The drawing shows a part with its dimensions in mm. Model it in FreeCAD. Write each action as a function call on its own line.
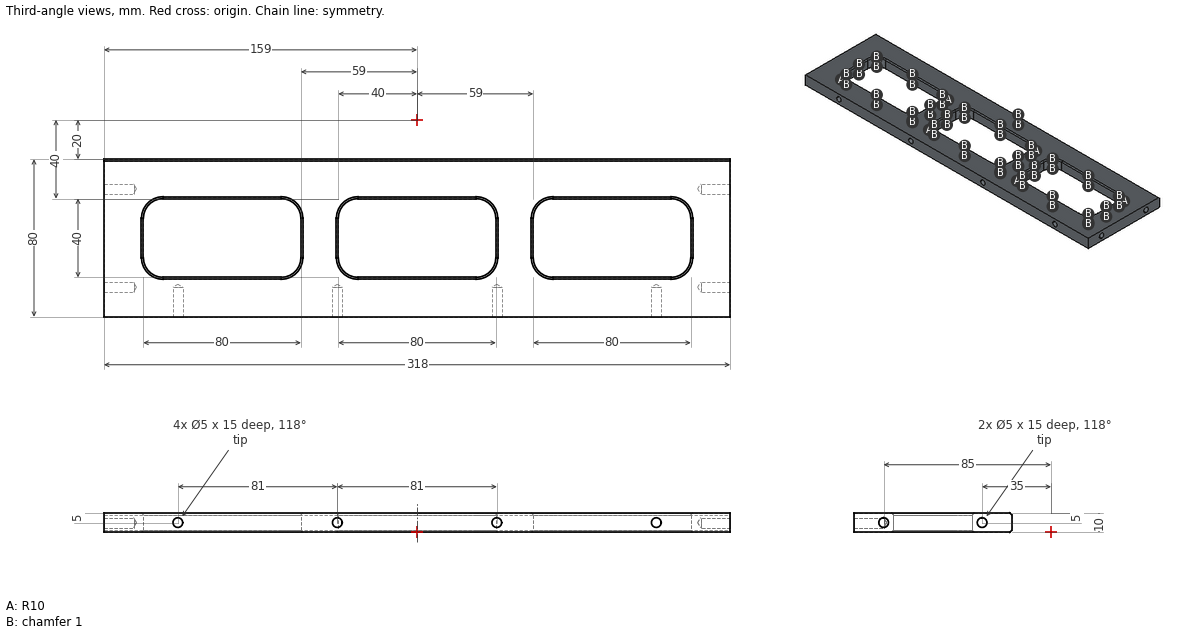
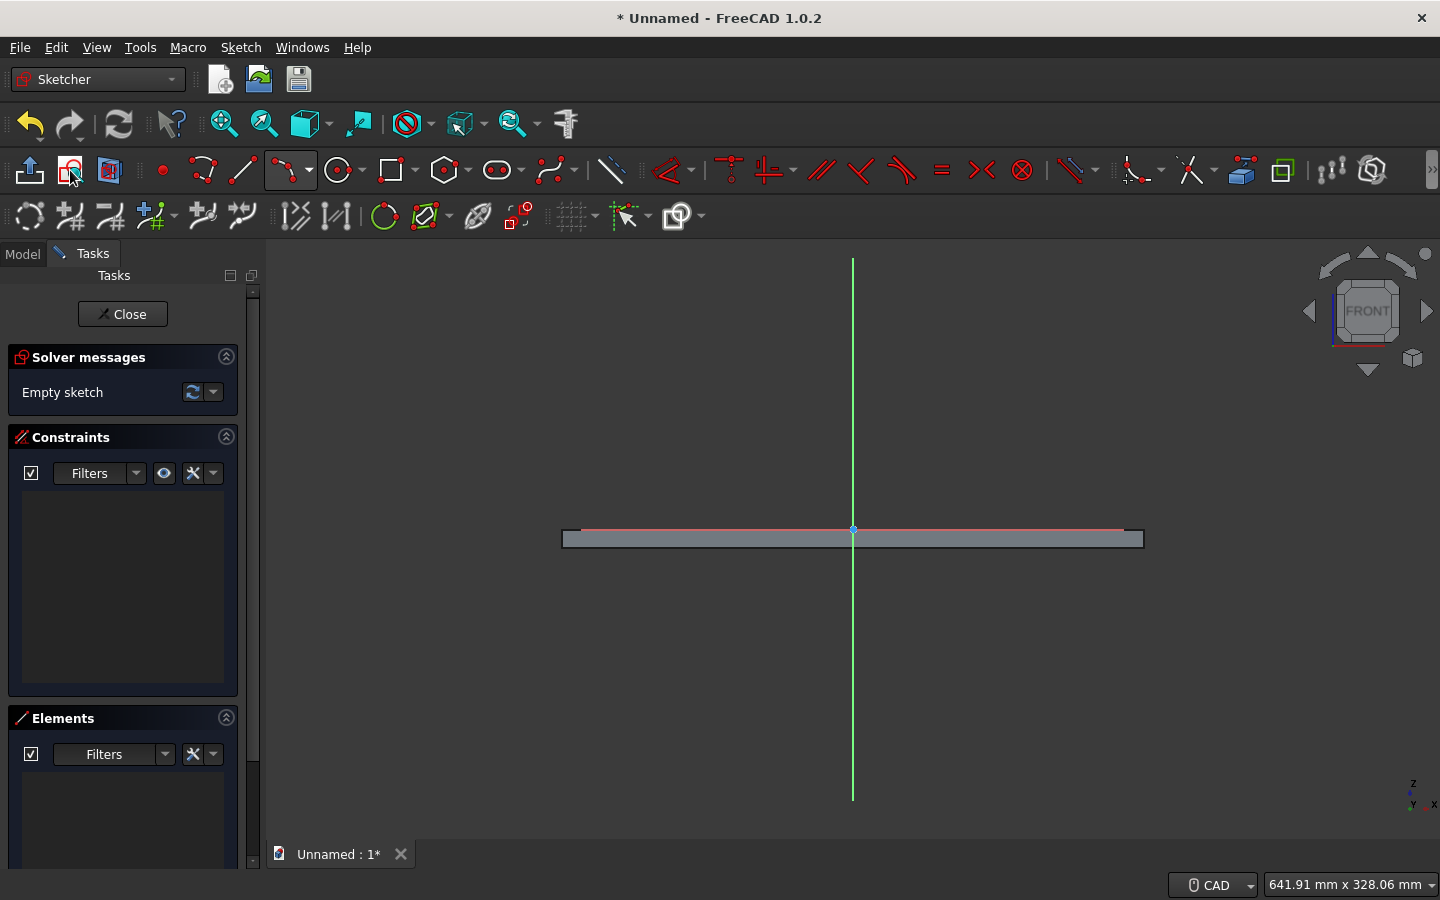
scroll(992, 532, up, 2)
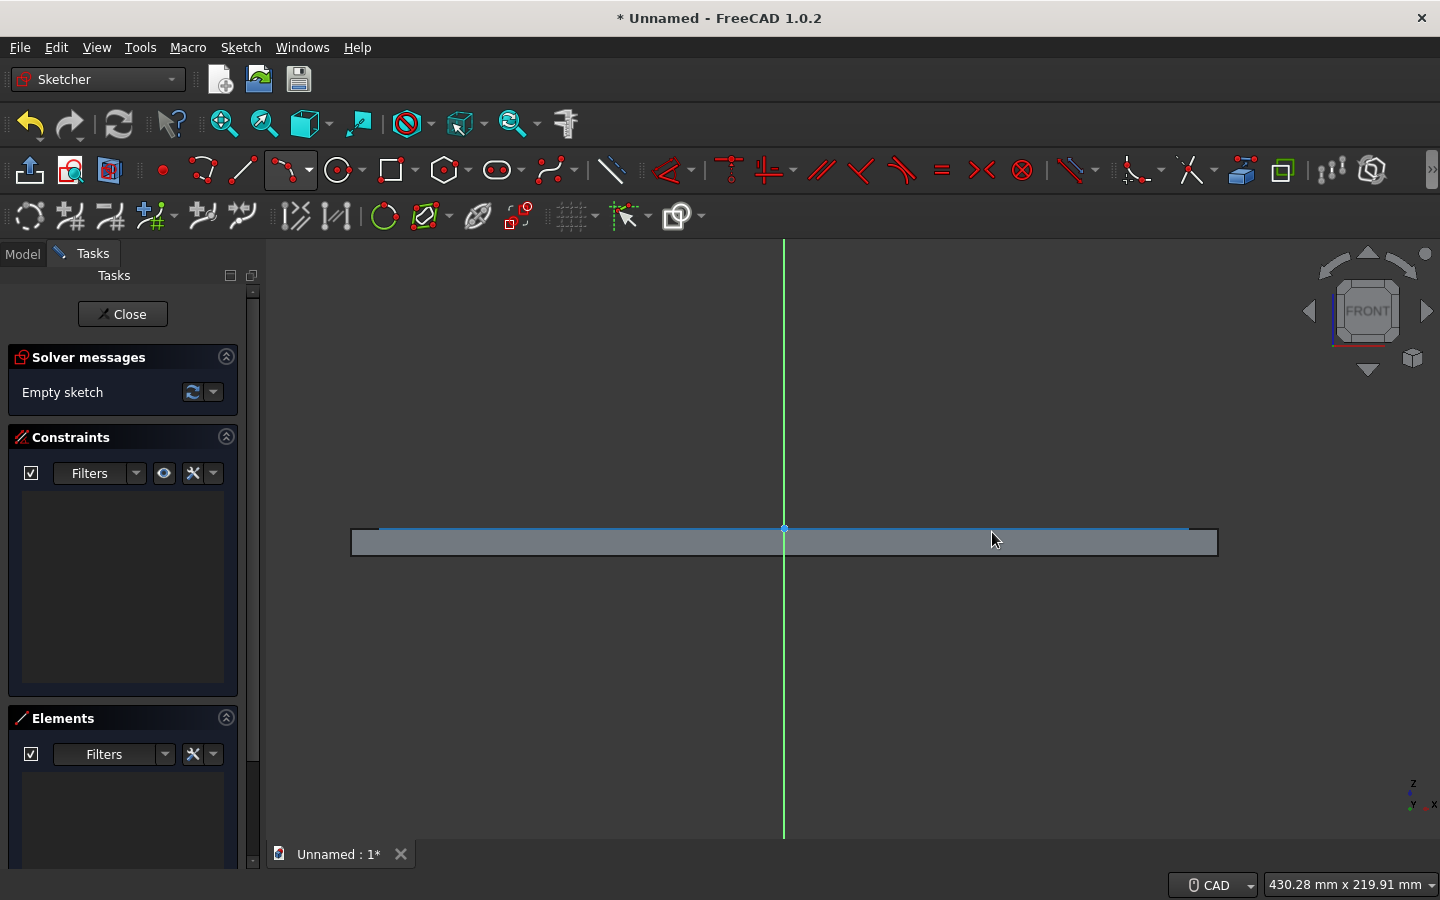
click(338, 170)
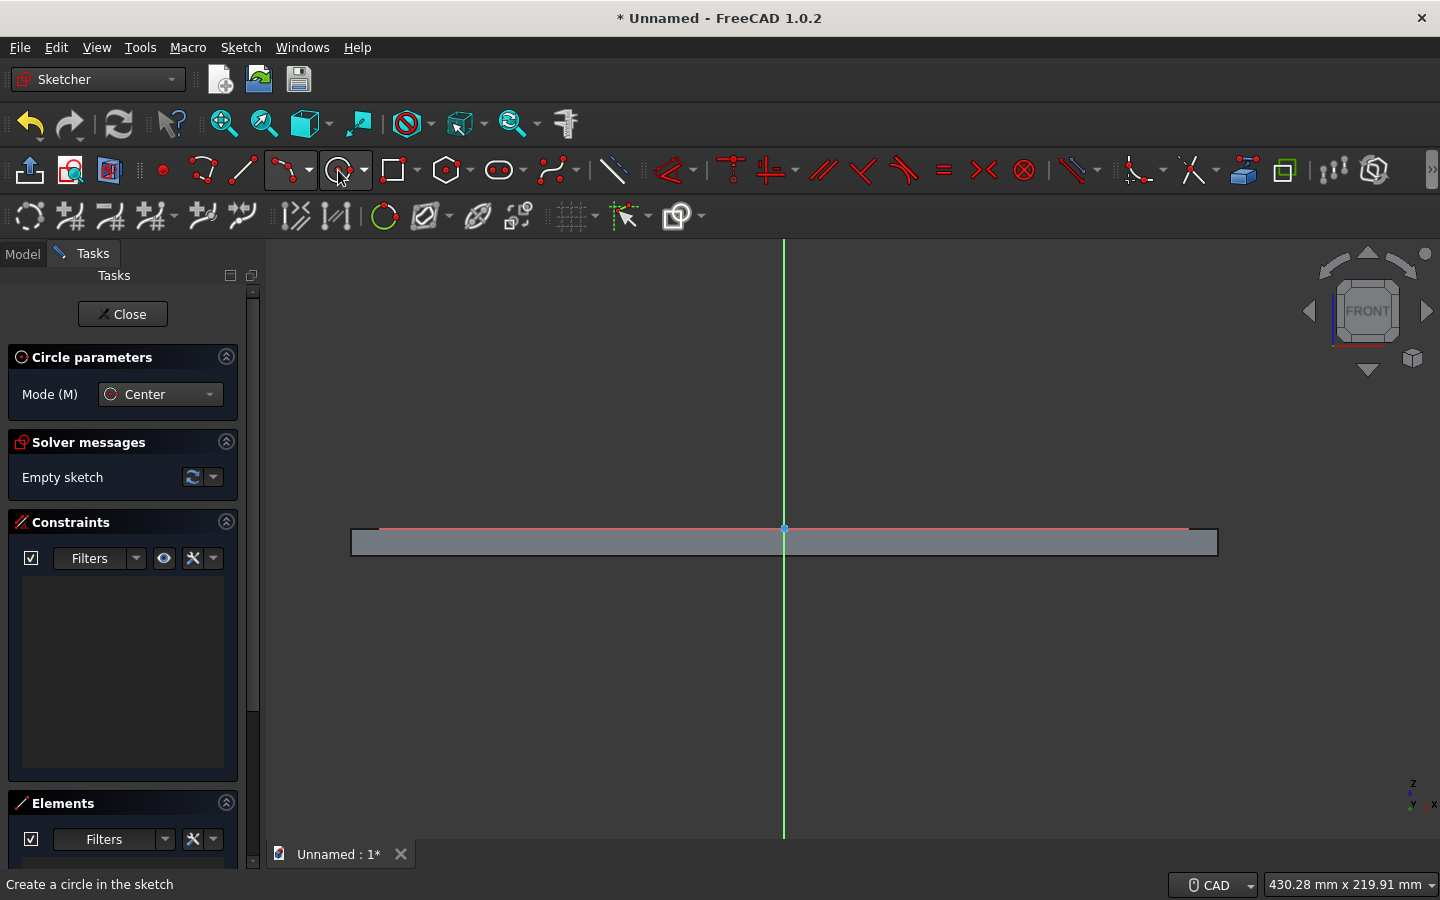
scroll(453, 542, up, 7)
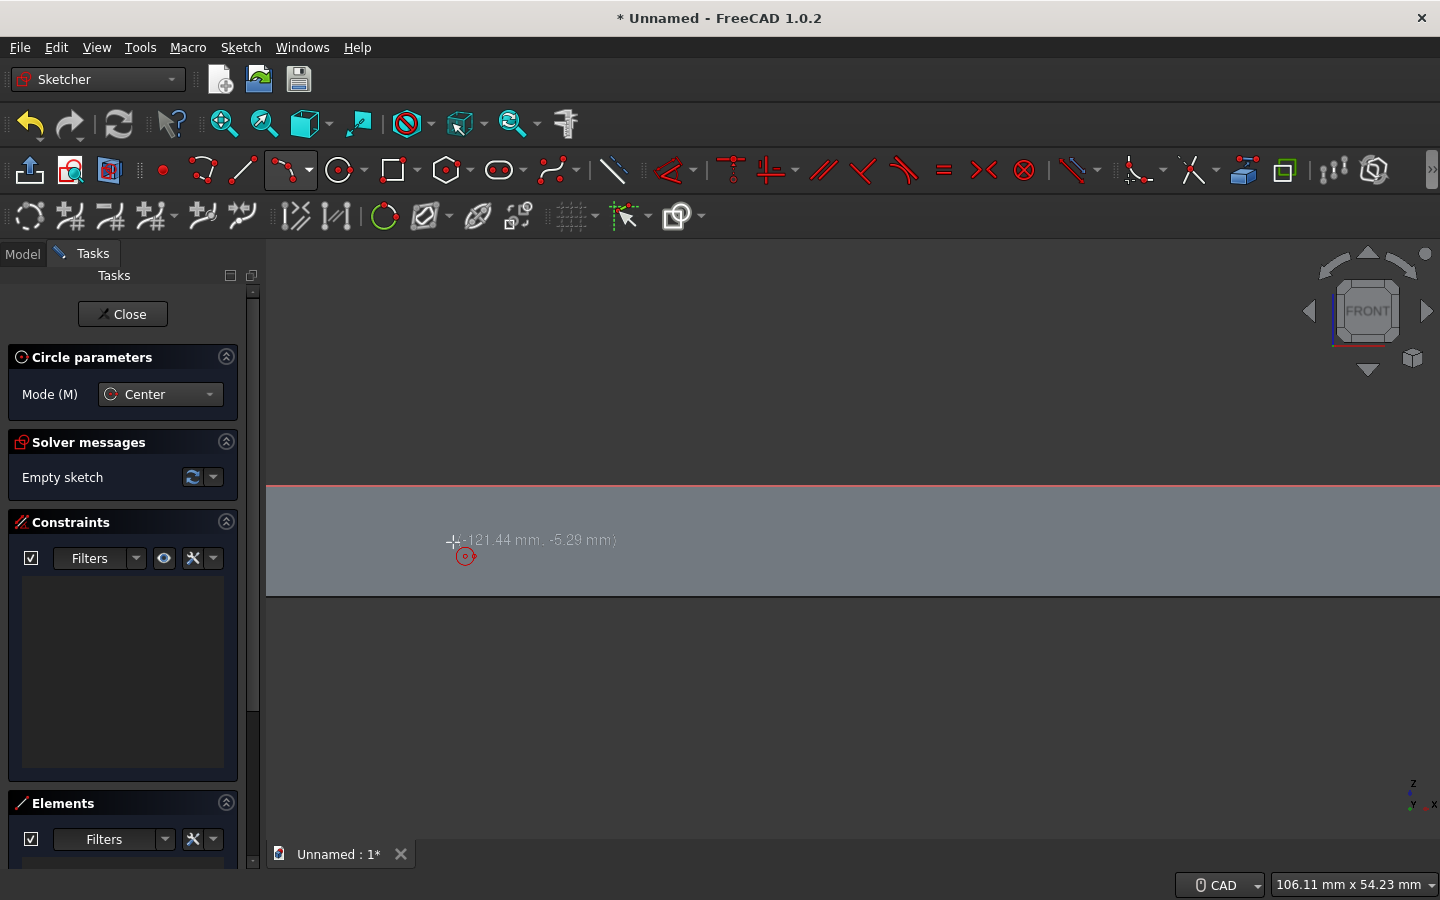
scroll(453, 543, down, 7)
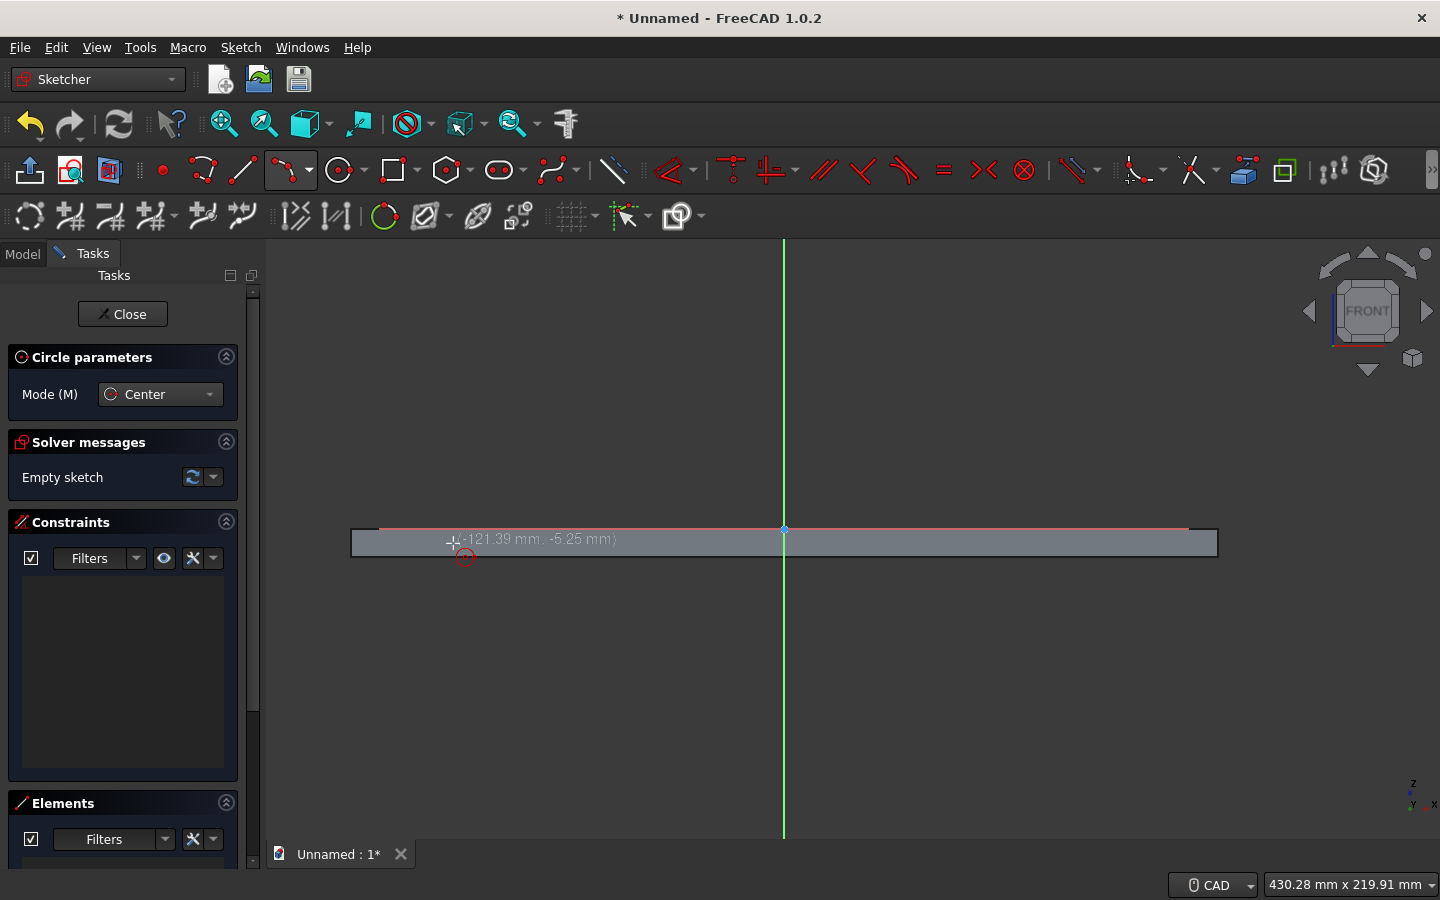
click(453, 543)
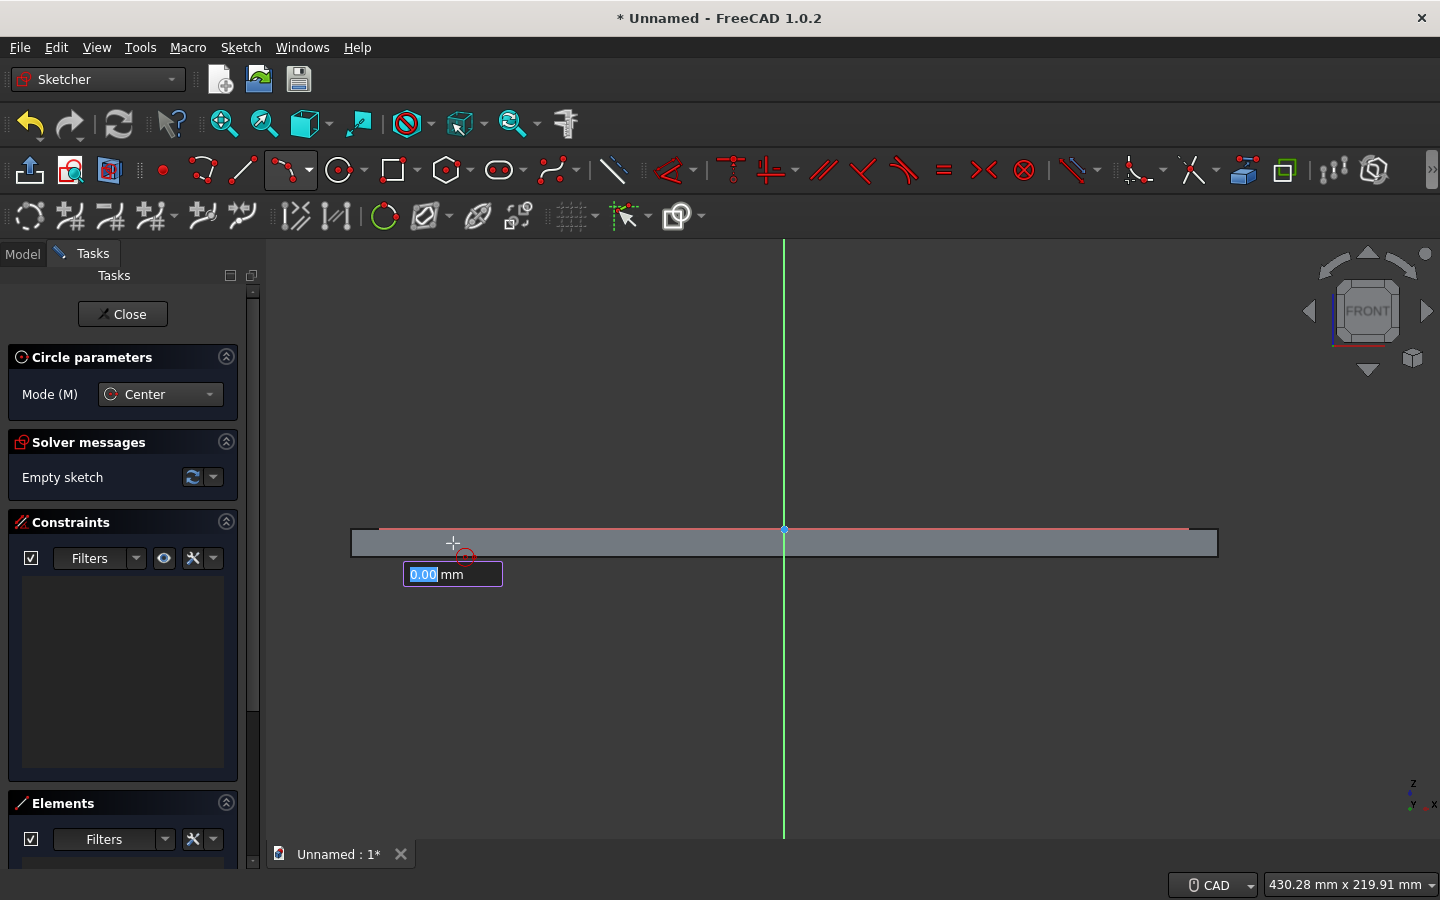
scroll(458, 548, up, 5)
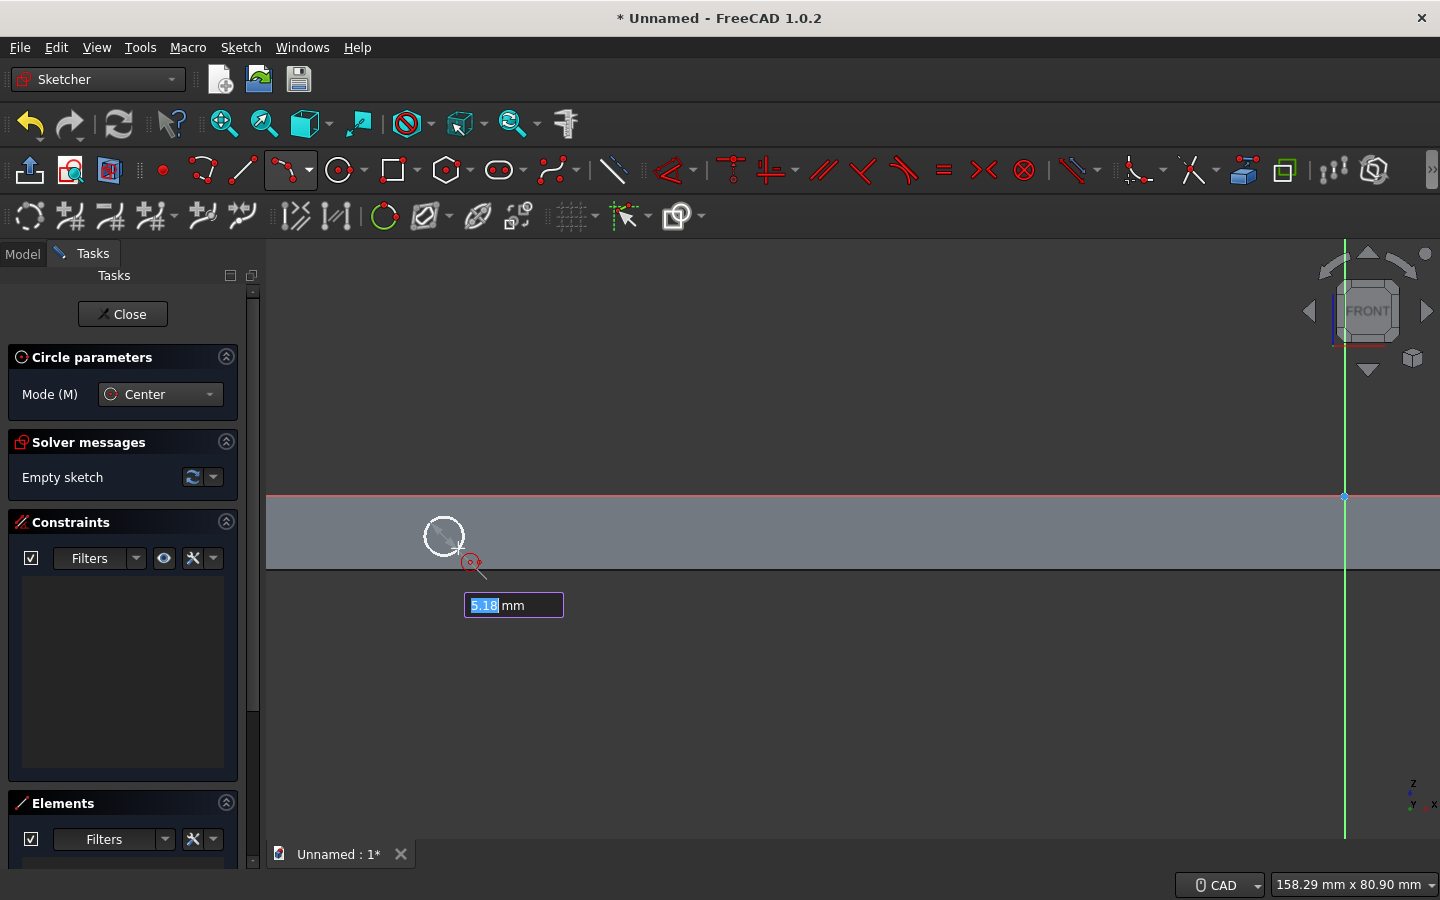
click(457, 547)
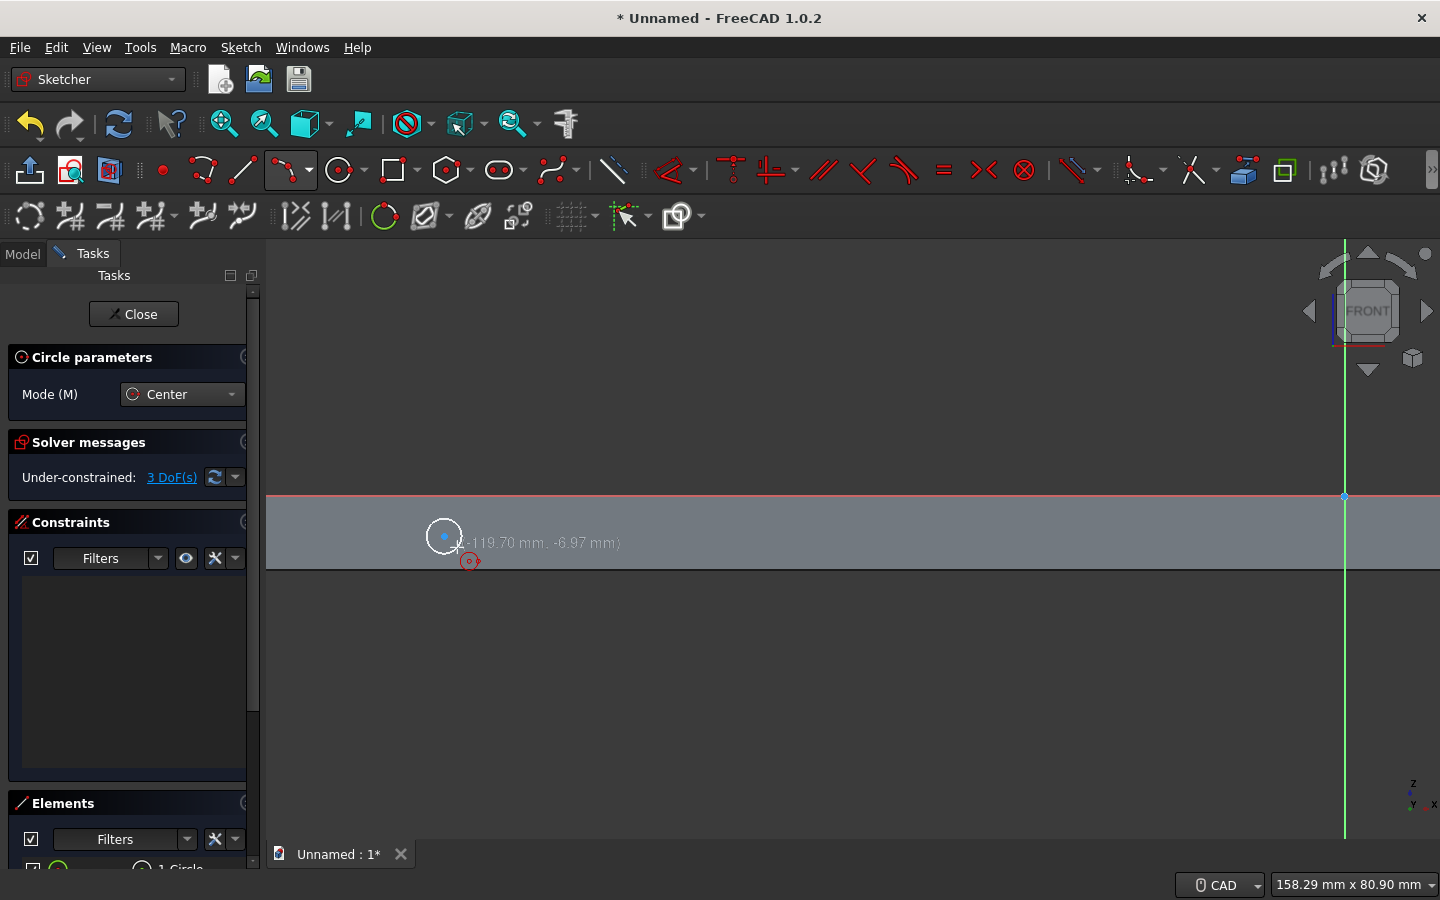
scroll(1044, 533, up, 2)